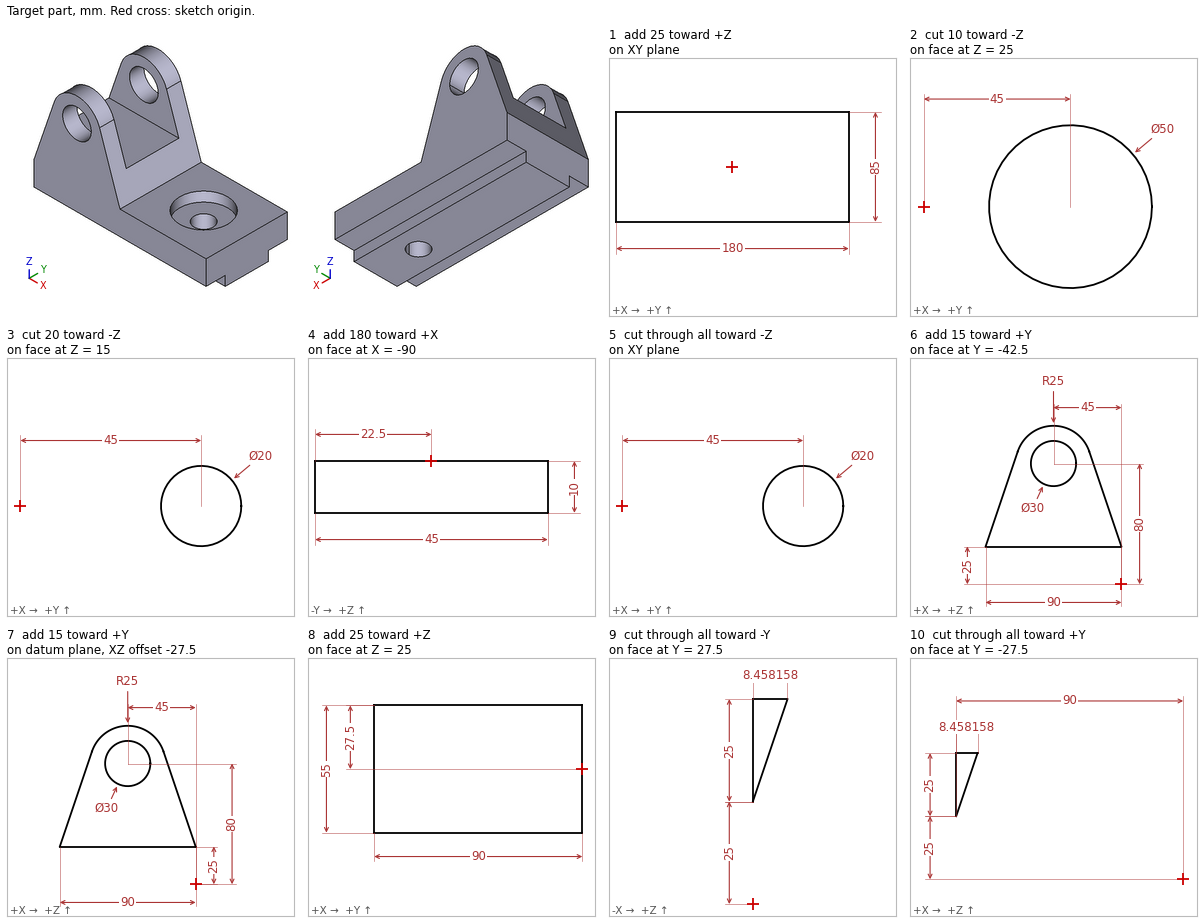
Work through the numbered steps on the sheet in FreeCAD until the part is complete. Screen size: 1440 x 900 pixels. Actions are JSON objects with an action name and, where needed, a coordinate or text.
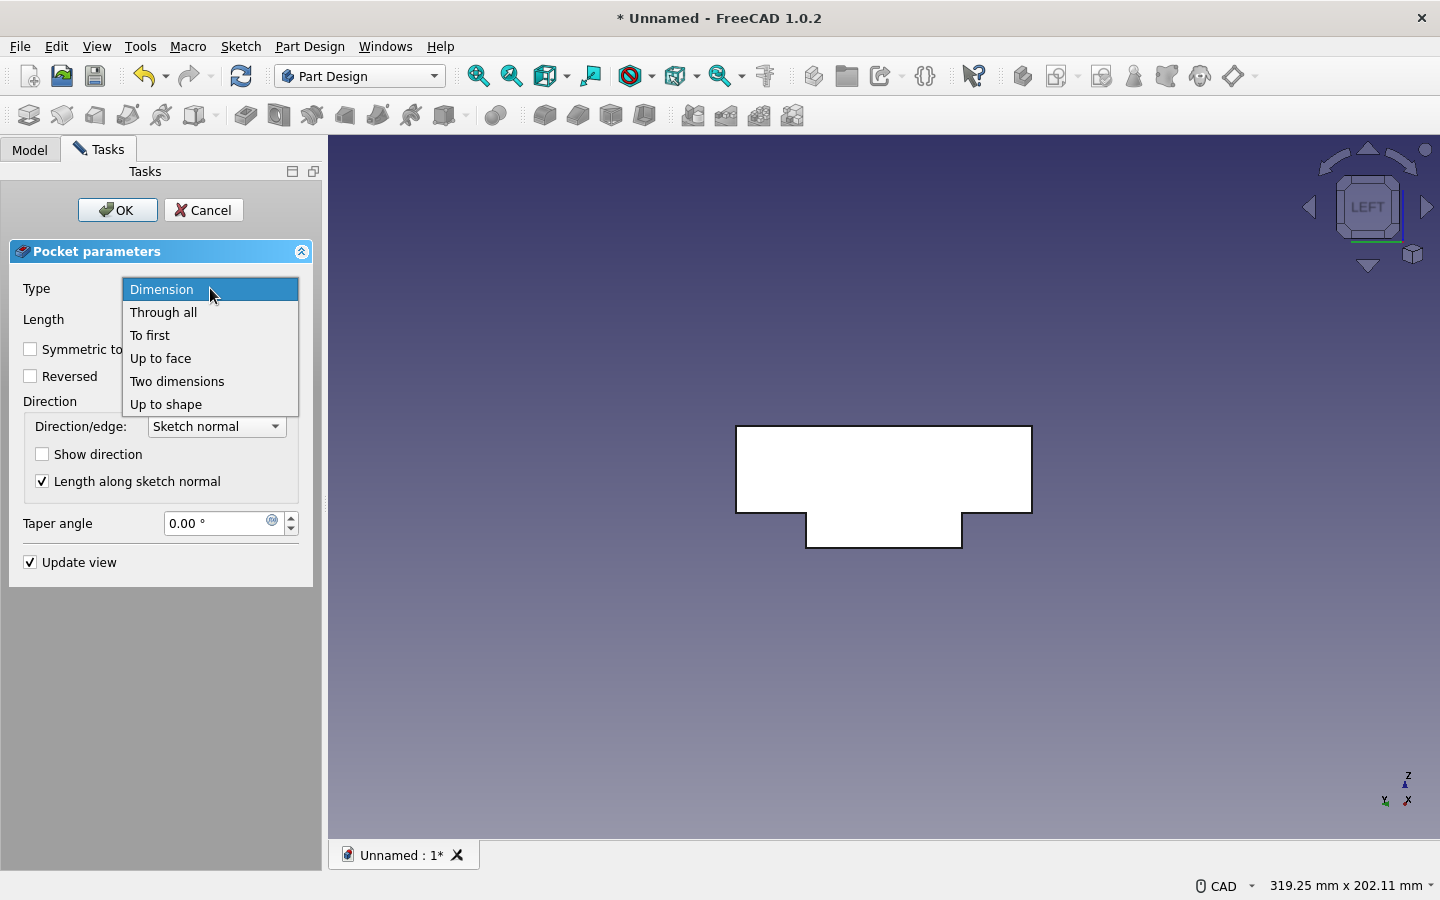
{"action": "left_click", "coordinate": [208, 312]}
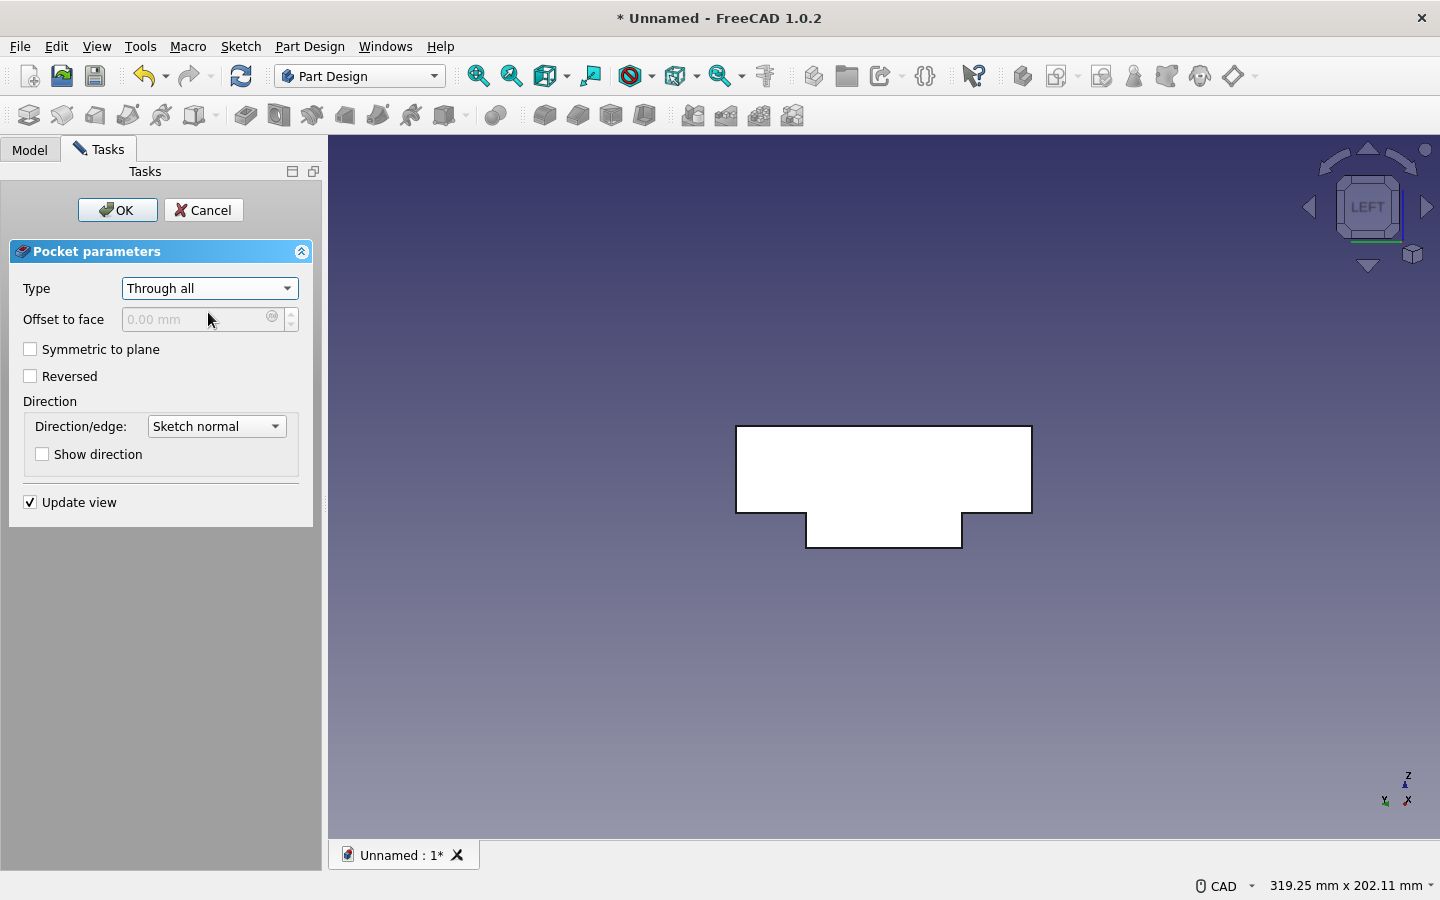
{"action": "left_click", "coordinate": [118, 210]}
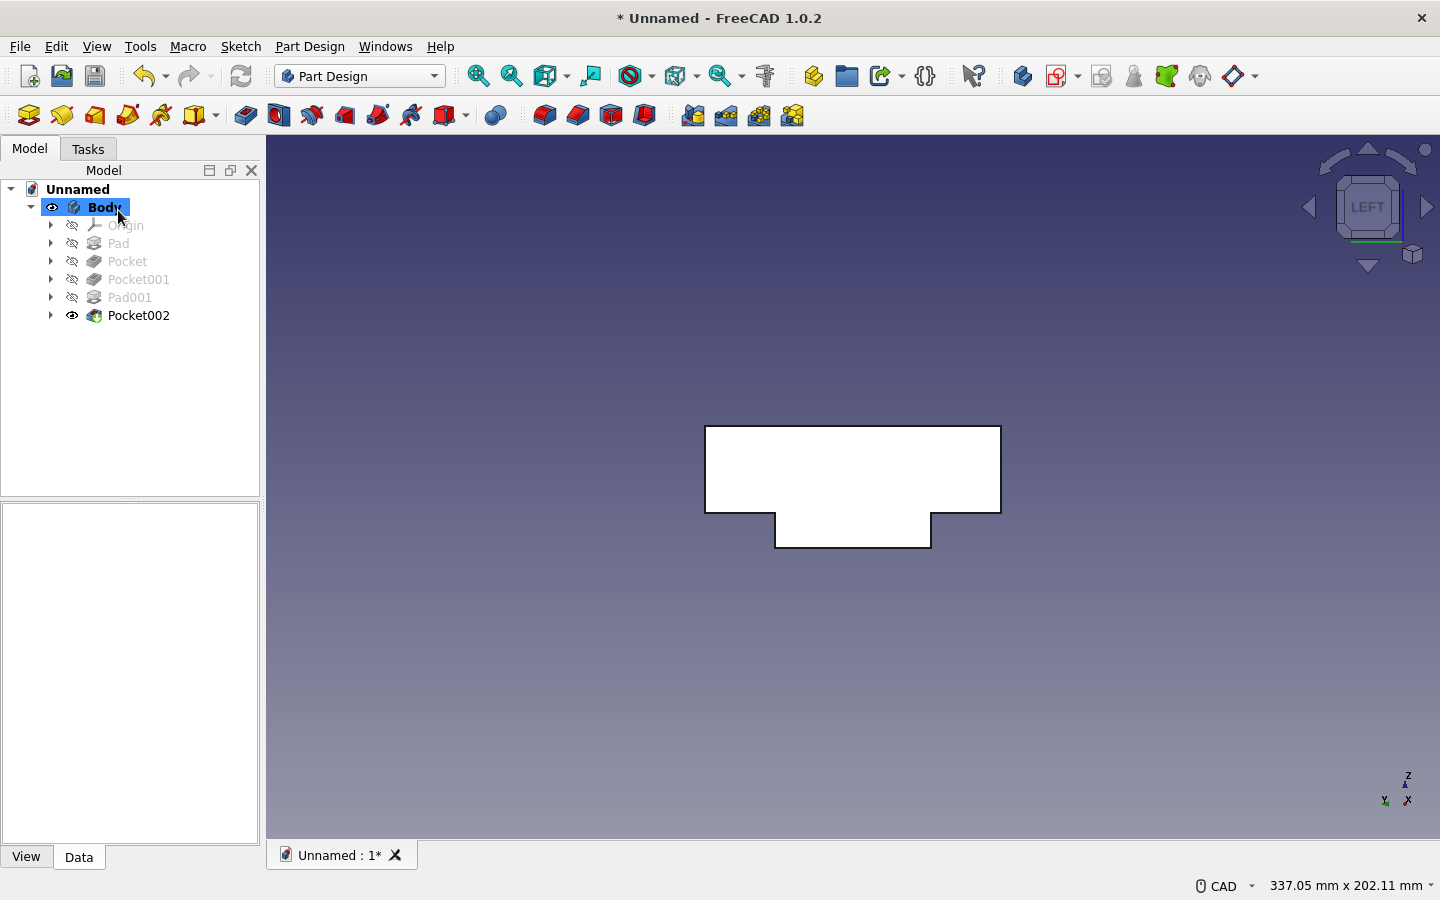
{"action": "left_click", "coordinate": [479, 76]}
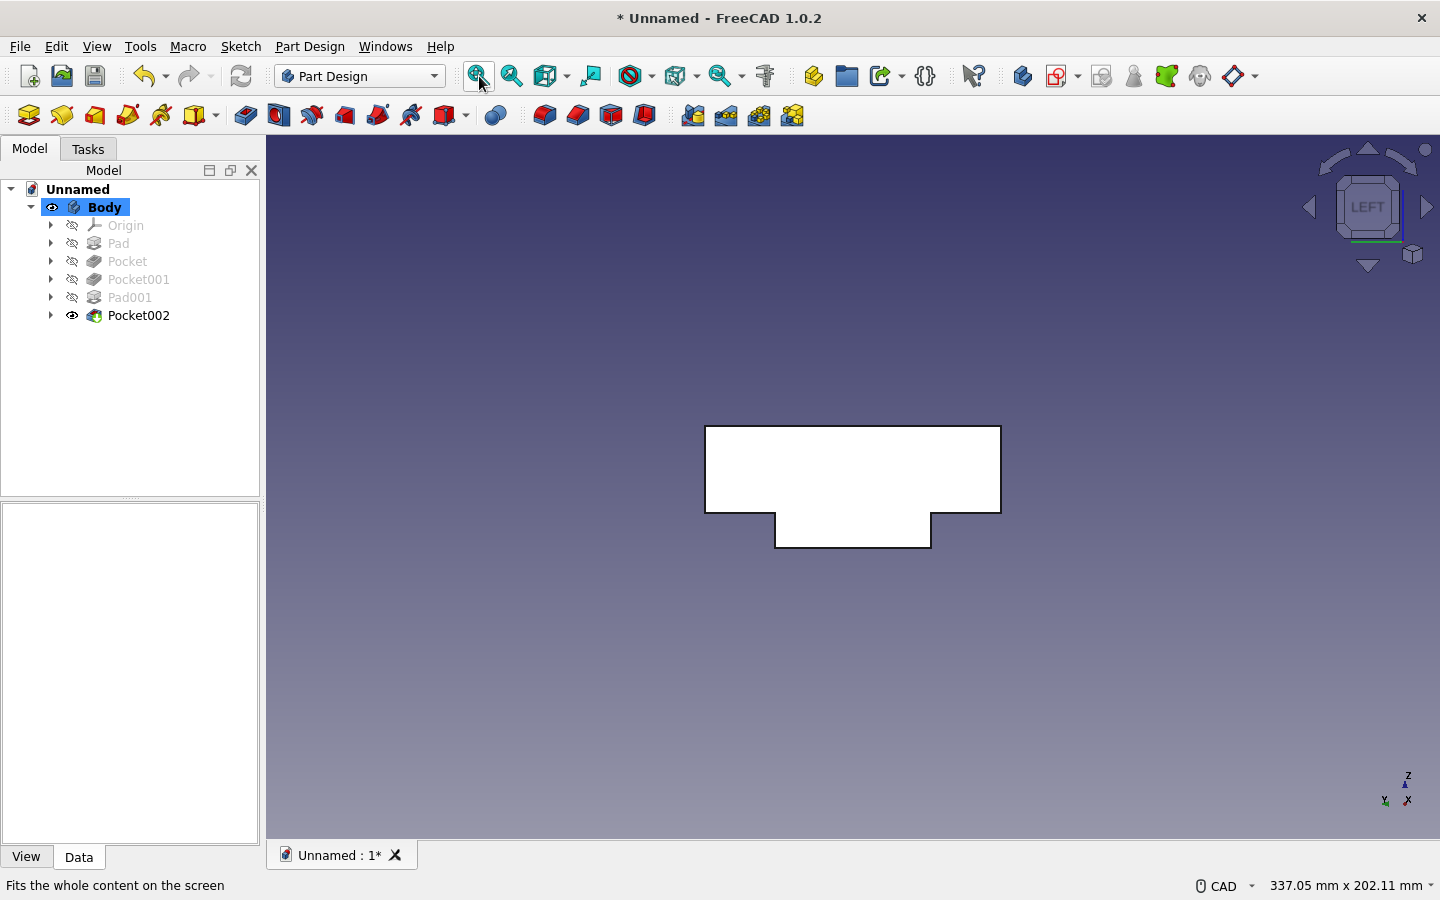
{"action": "key", "text": "0"}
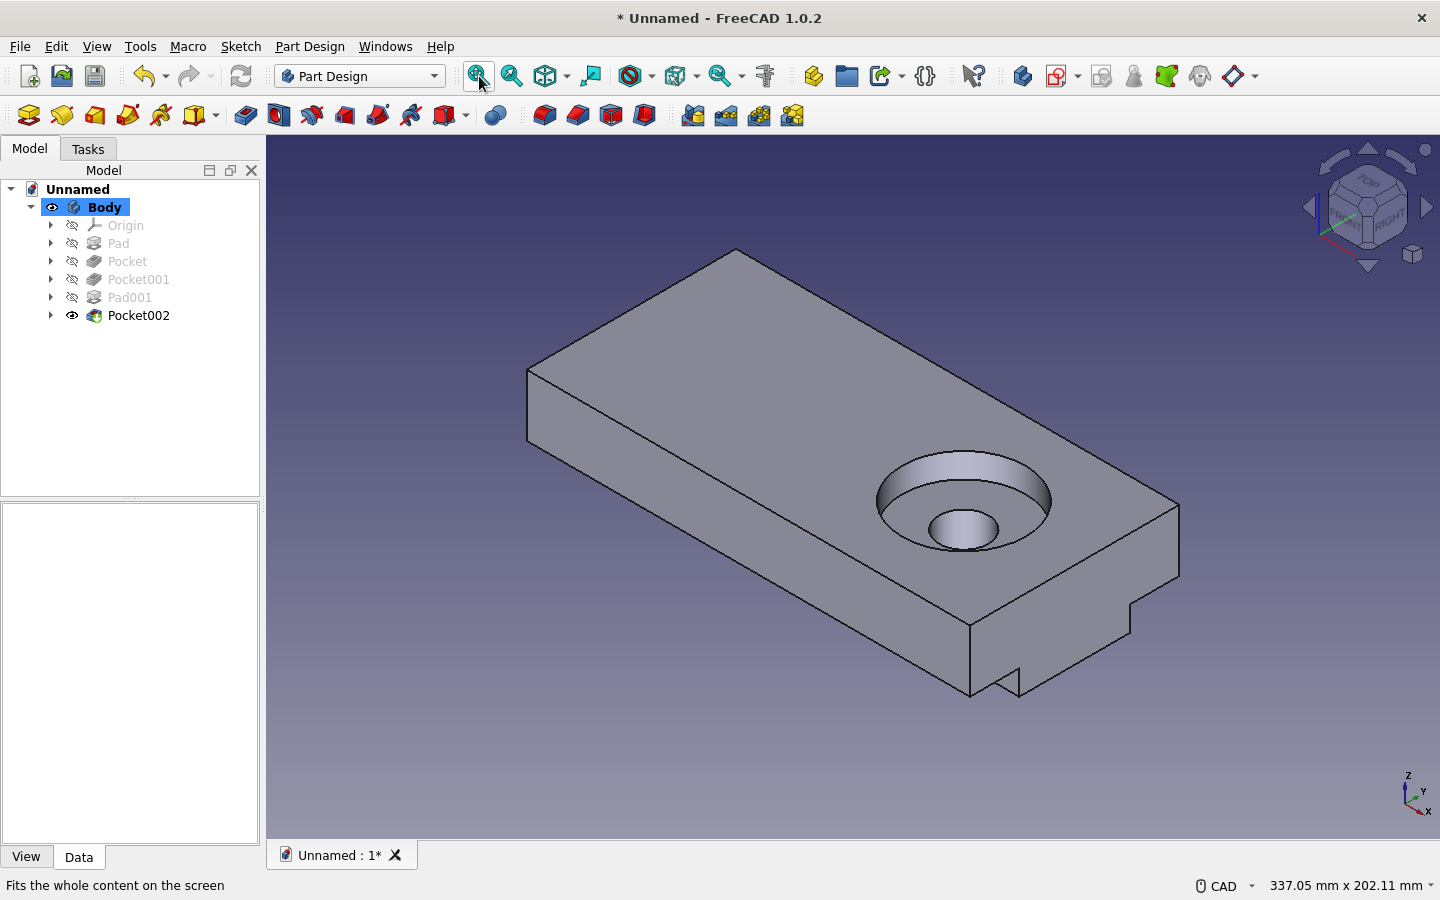
{"action": "left_click", "coordinate": [938, 642]}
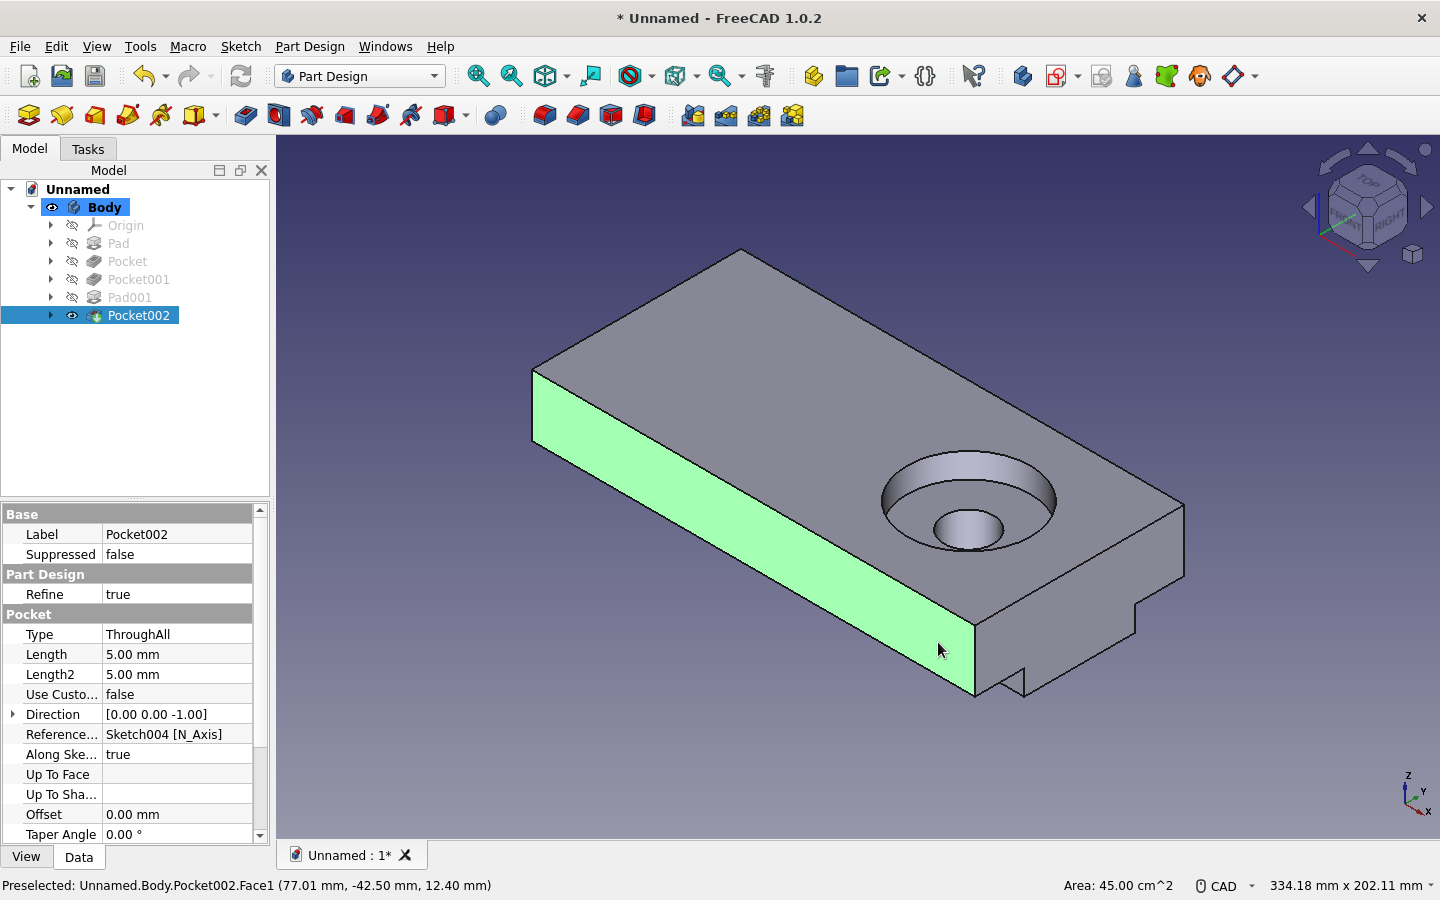
{"action": "left_click", "coordinate": [1056, 76]}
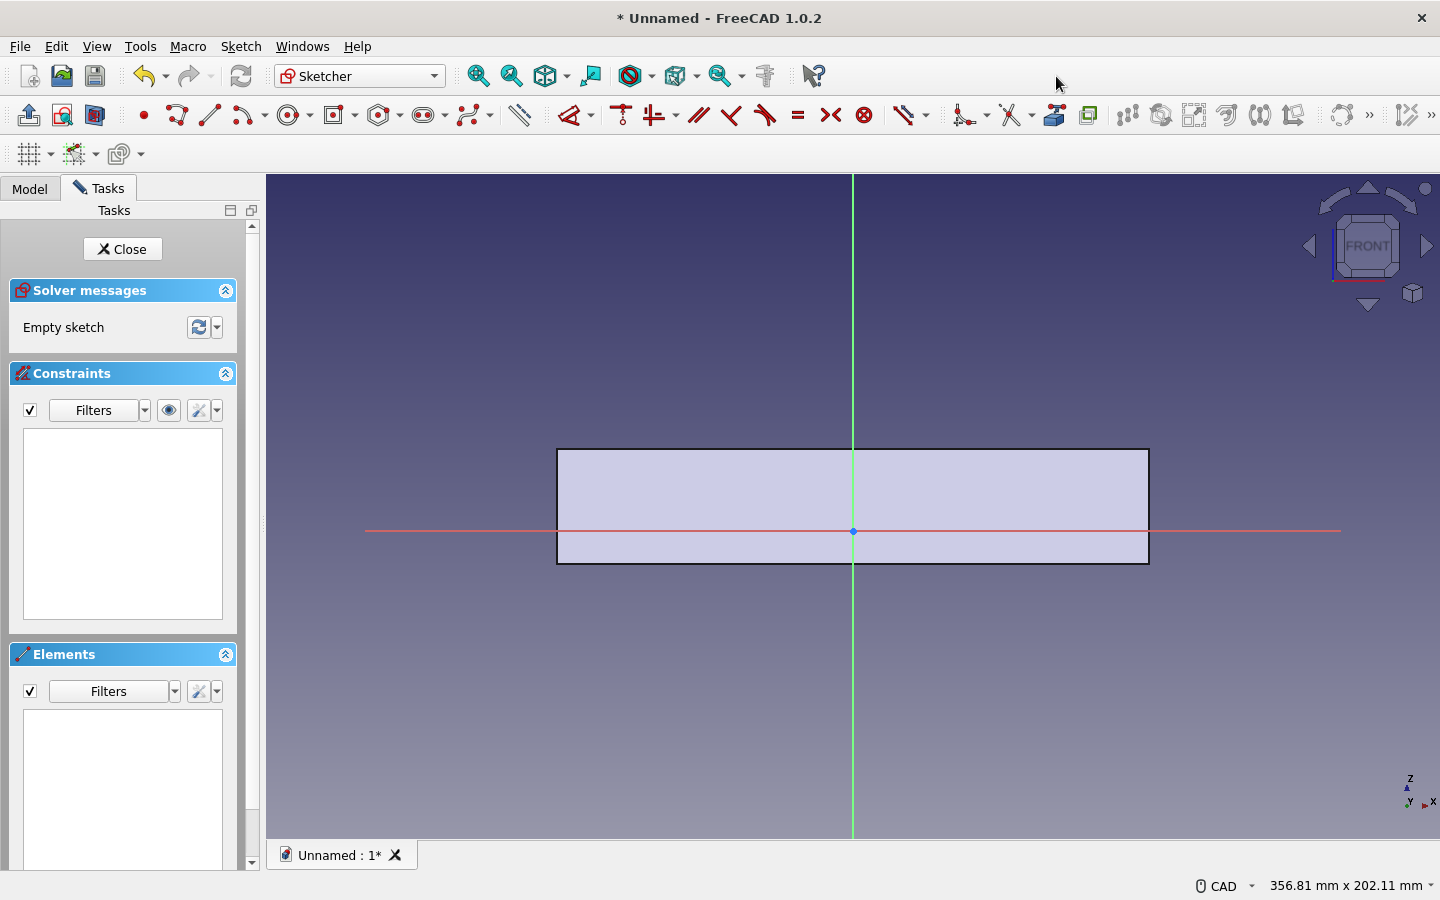
{"action": "scroll", "coordinate": [1144, 811], "scroll_direction": "down", "scroll_amount": 1}